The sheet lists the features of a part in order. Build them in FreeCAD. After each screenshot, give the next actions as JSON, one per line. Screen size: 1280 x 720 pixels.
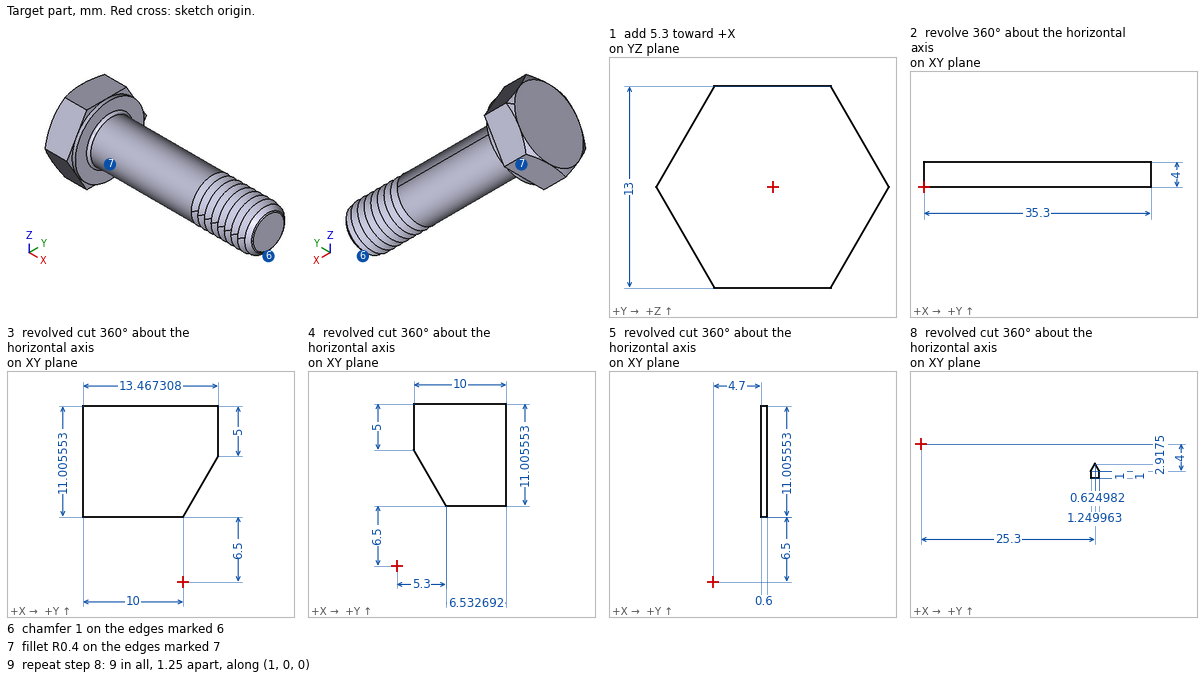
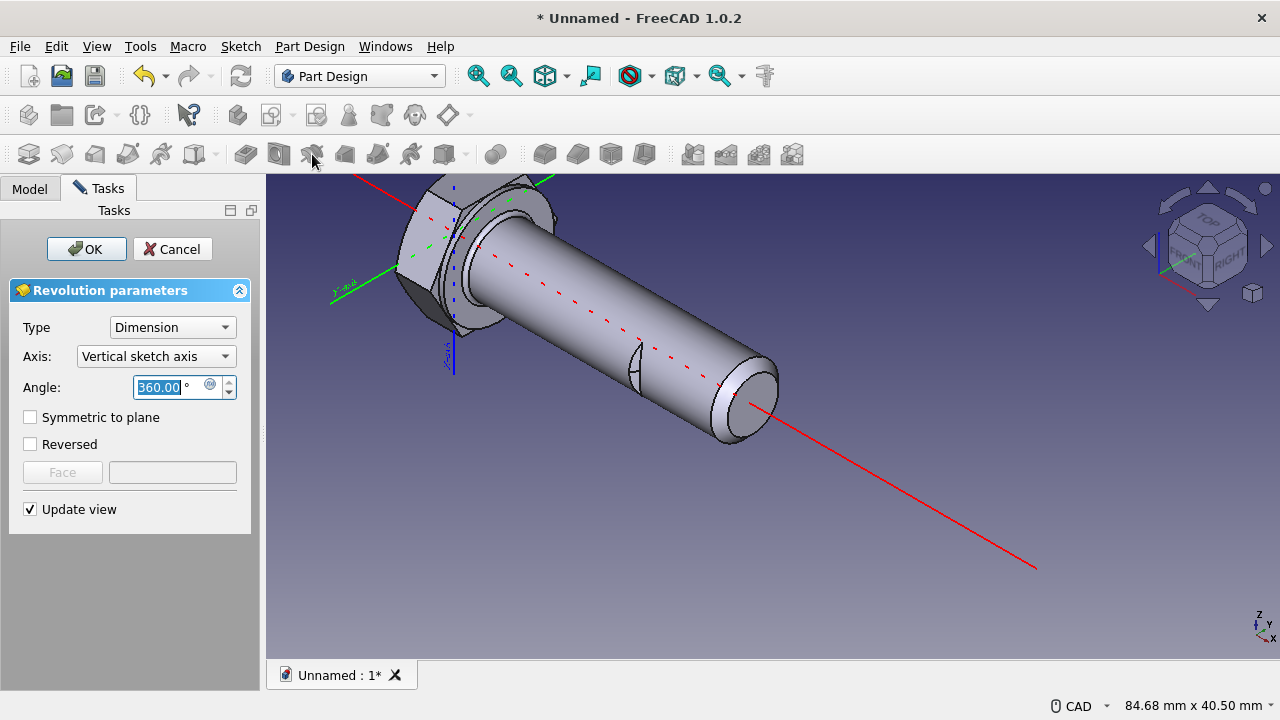
{"action": "left_click", "coordinate": [157, 356]}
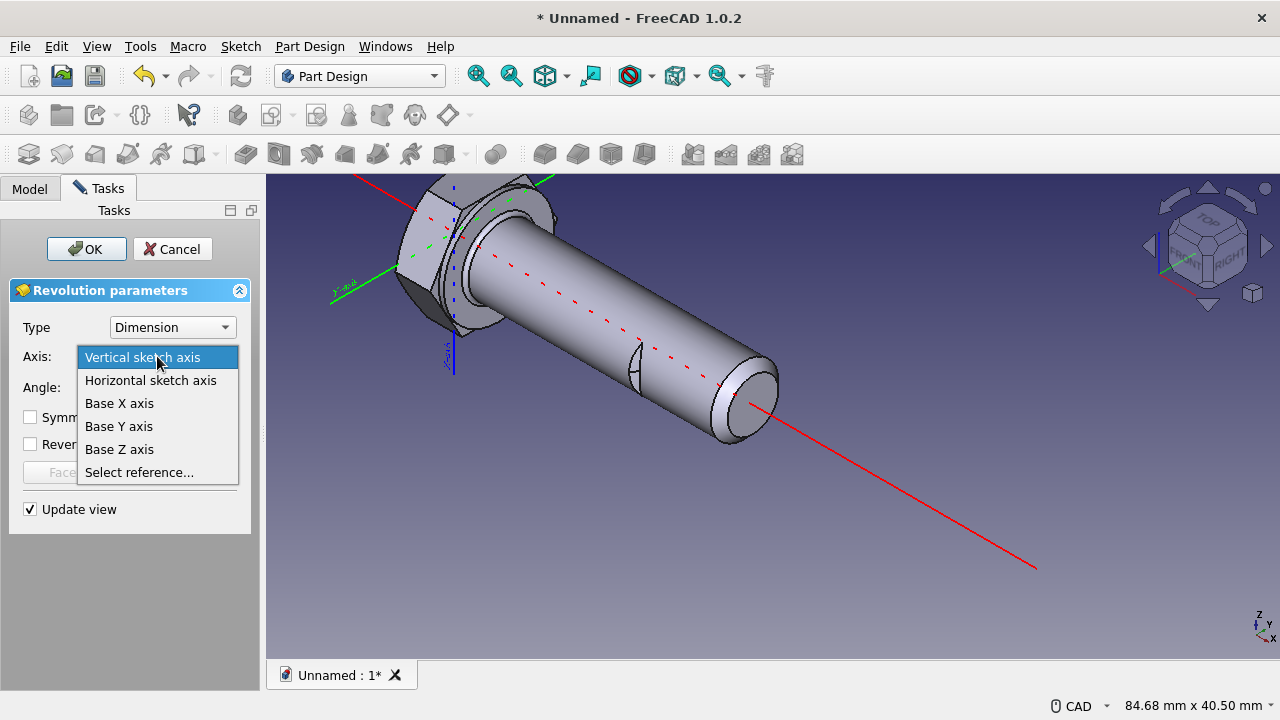
{"action": "left_click", "coordinate": [156, 380]}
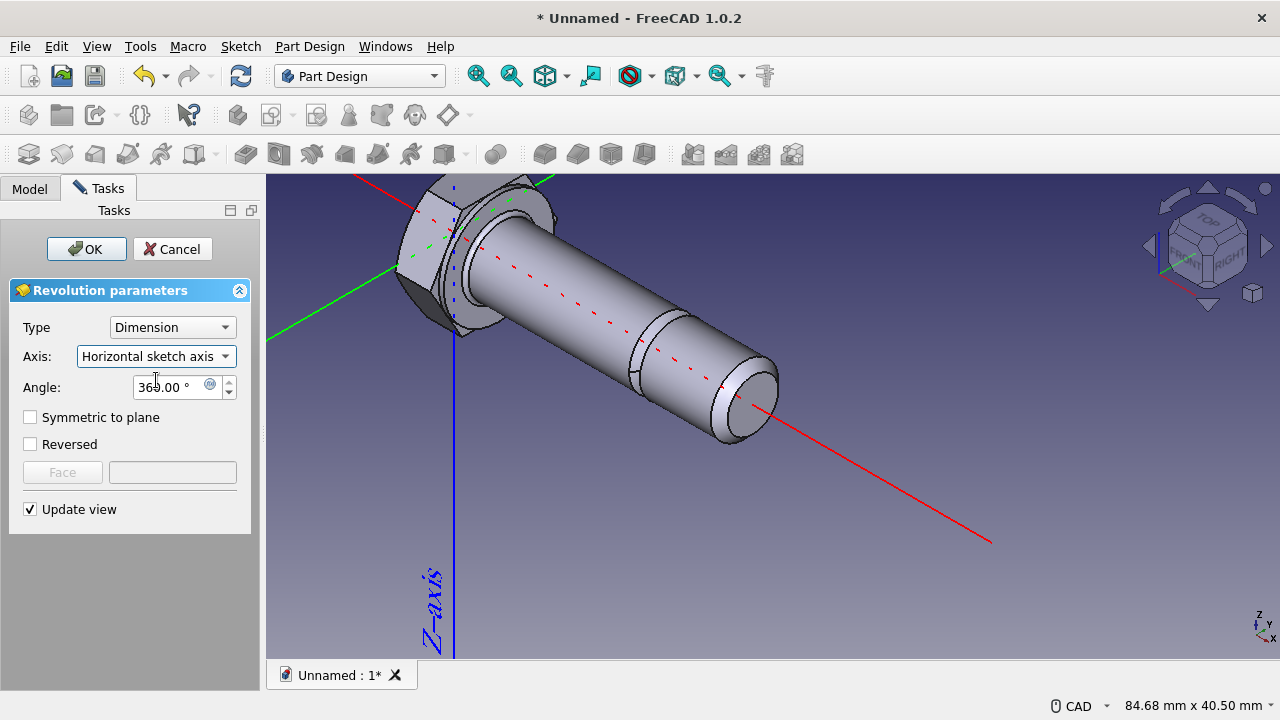
{"action": "left_click", "coordinate": [87, 249]}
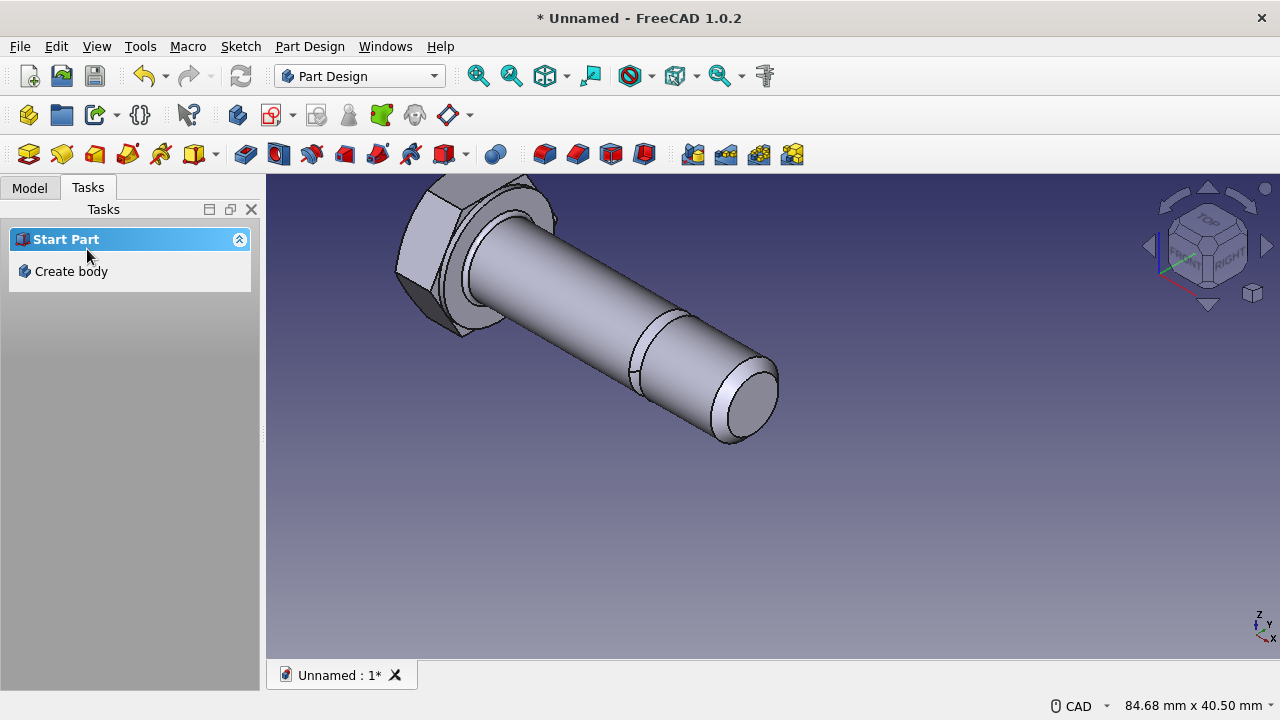
{"action": "key", "text": "v f"}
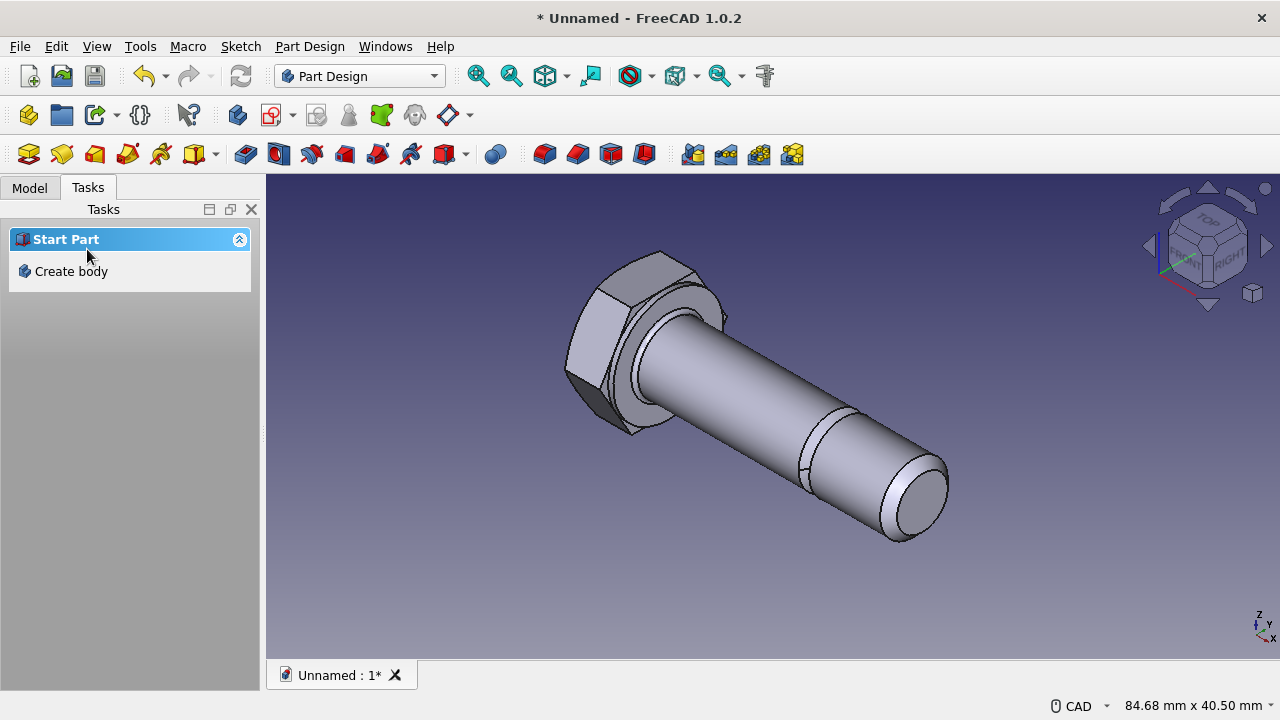
{"action": "left_click", "coordinate": [30, 188]}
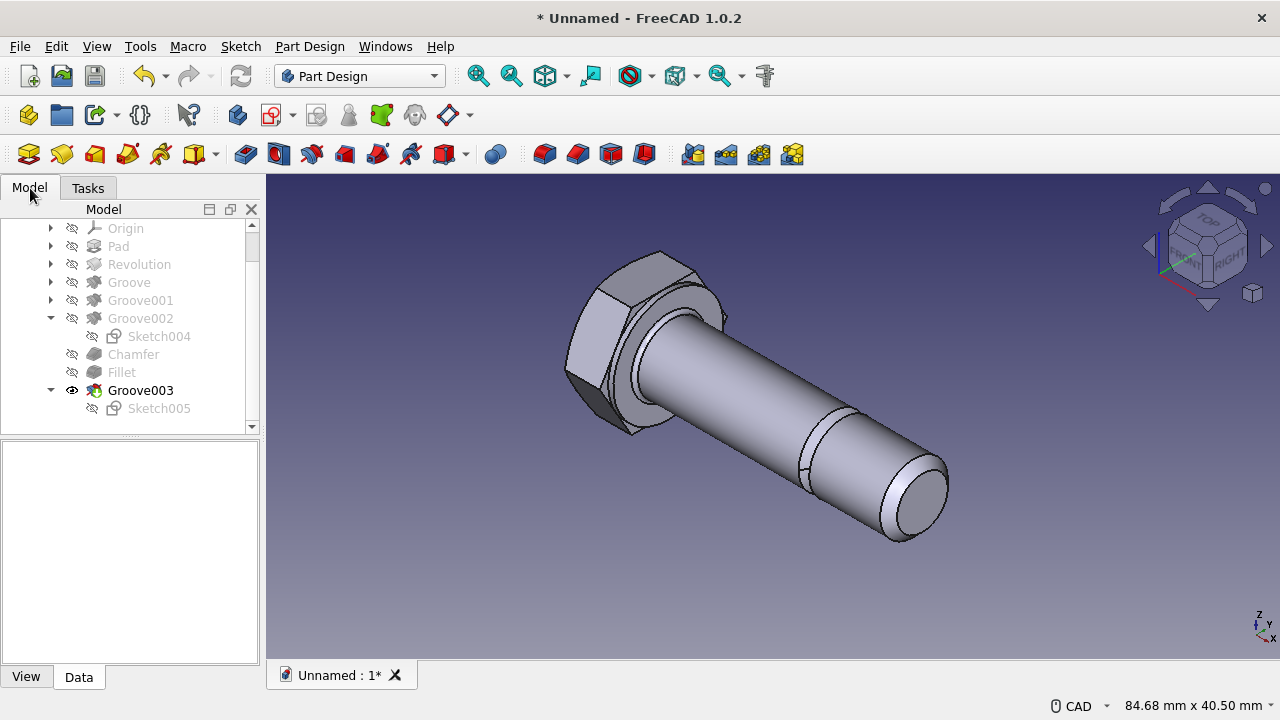
{"action": "left_click", "coordinate": [117, 390]}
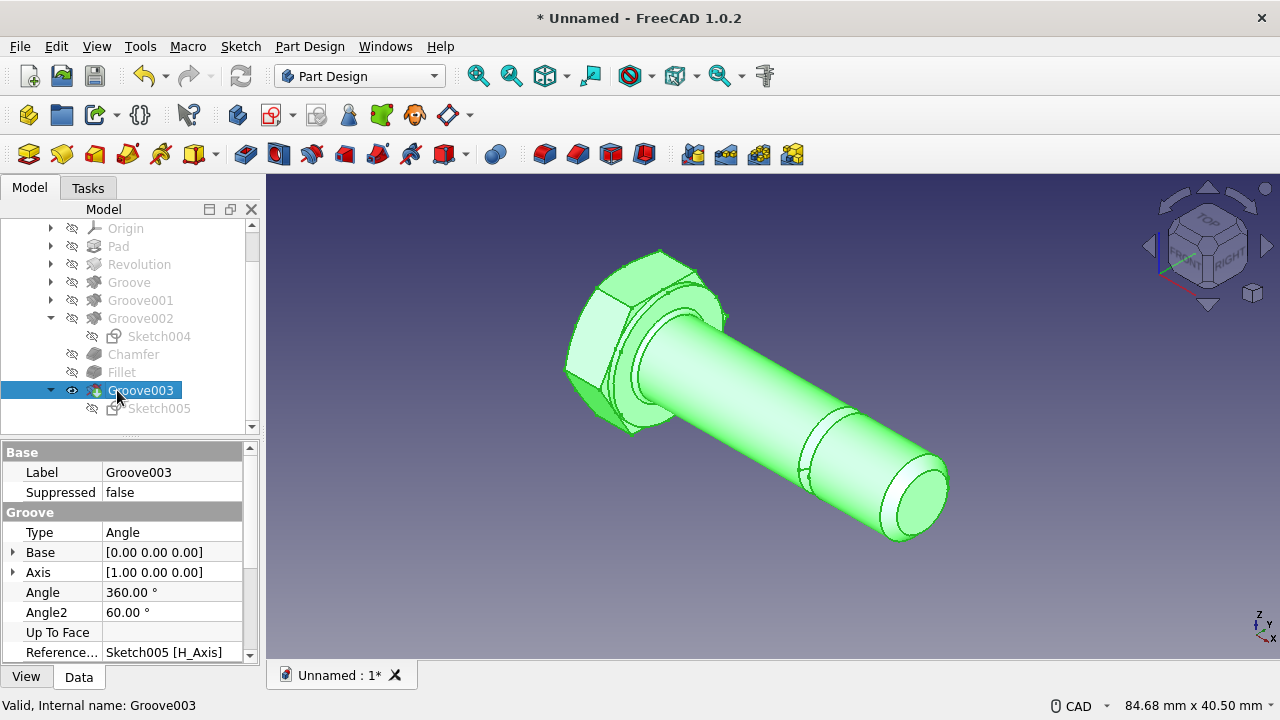
{"action": "left_click", "coordinate": [726, 154]}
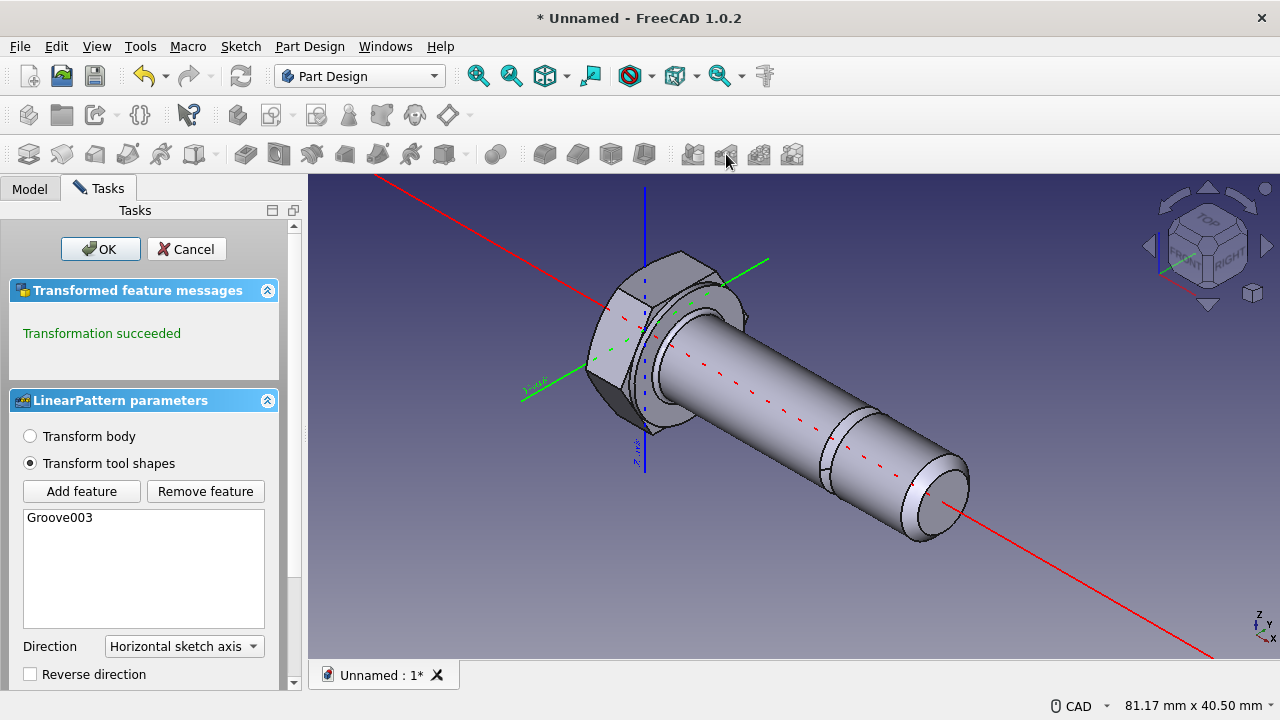
{"action": "left_click", "coordinate": [185, 646]}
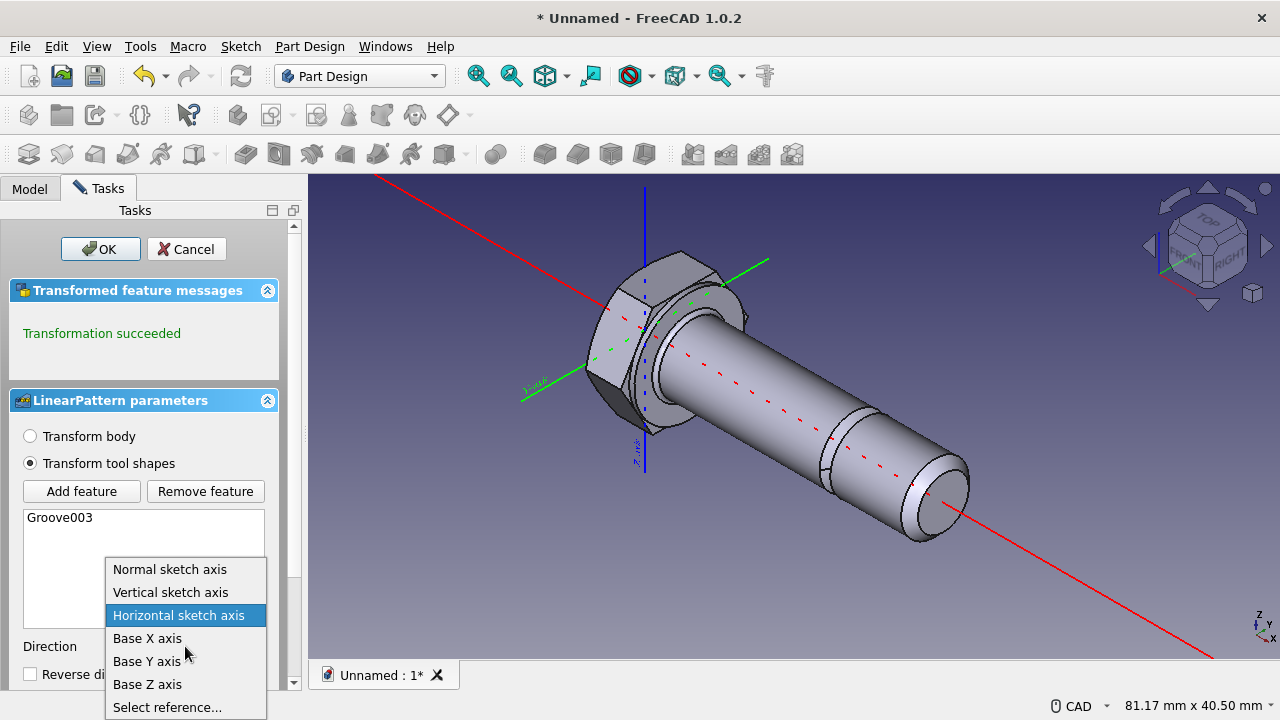
{"action": "left_click", "coordinate": [184, 638]}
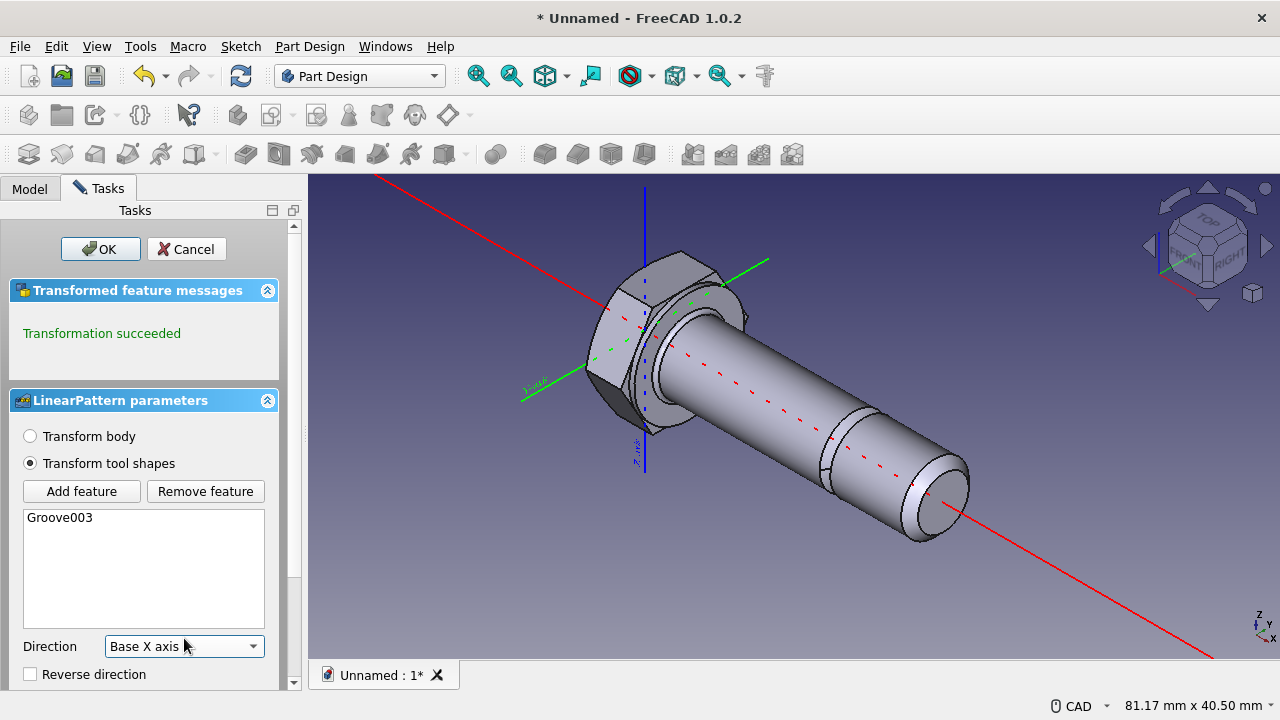
{"action": "scroll", "coordinate": [294, 455], "scroll_direction": "down", "scroll_amount": 2}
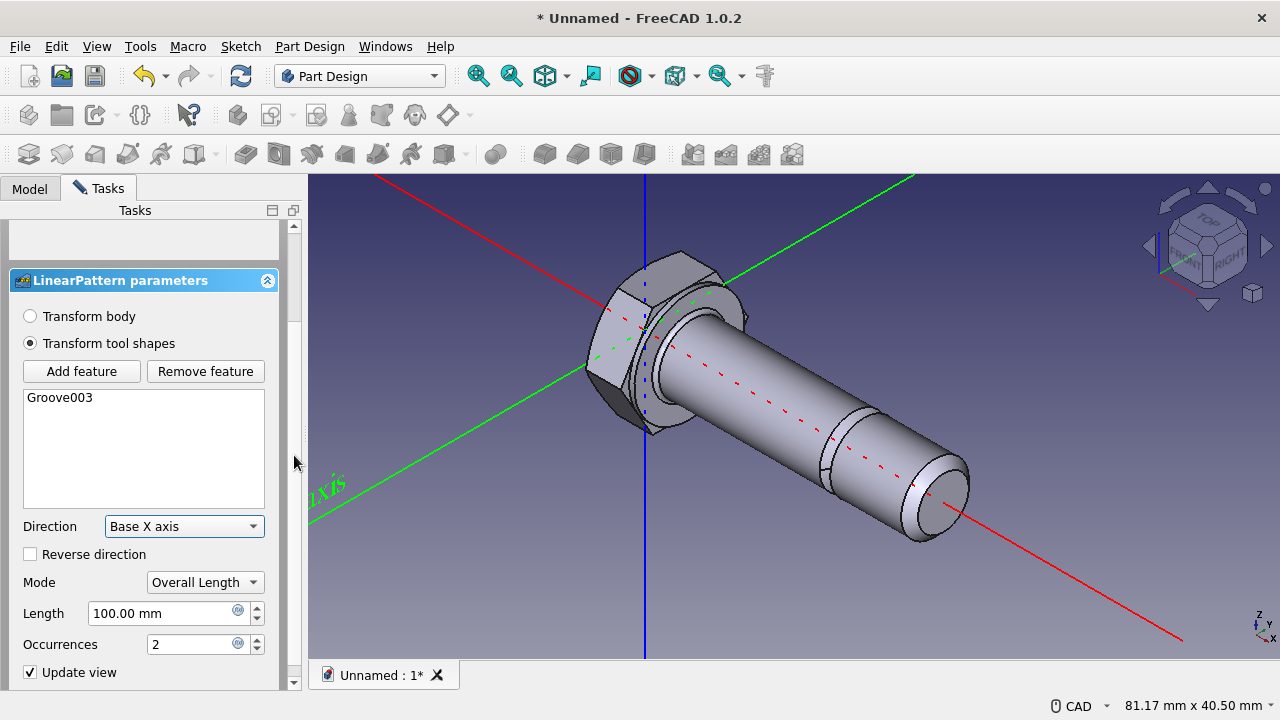
{"action": "left_click", "coordinate": [206, 582]}